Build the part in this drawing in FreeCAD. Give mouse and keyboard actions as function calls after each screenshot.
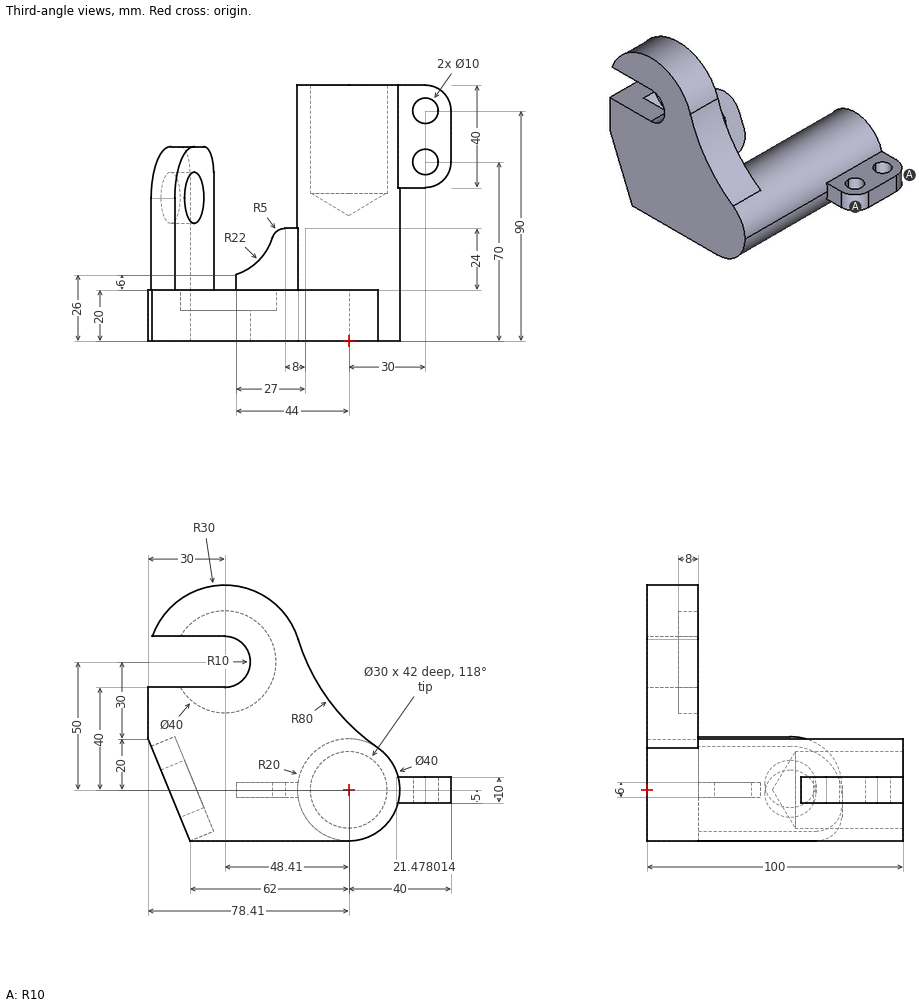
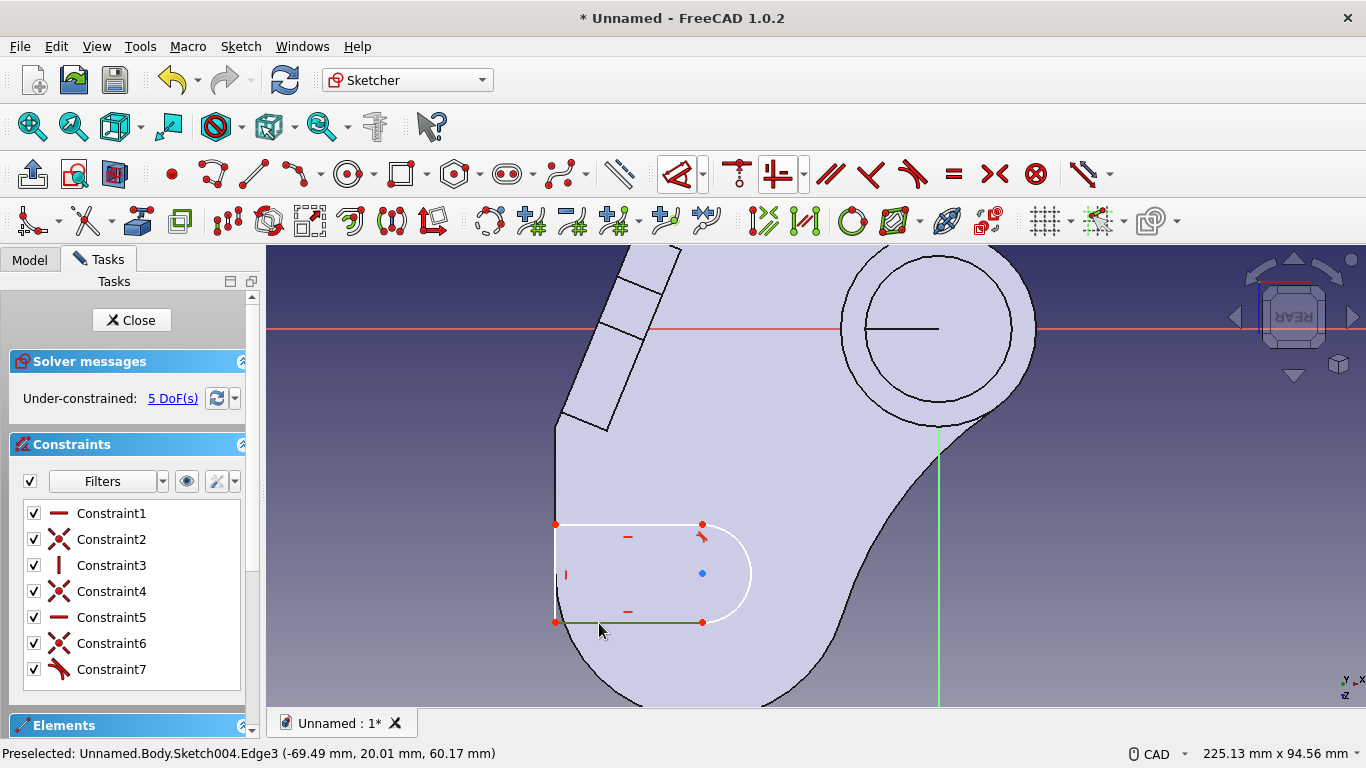
click(742, 603)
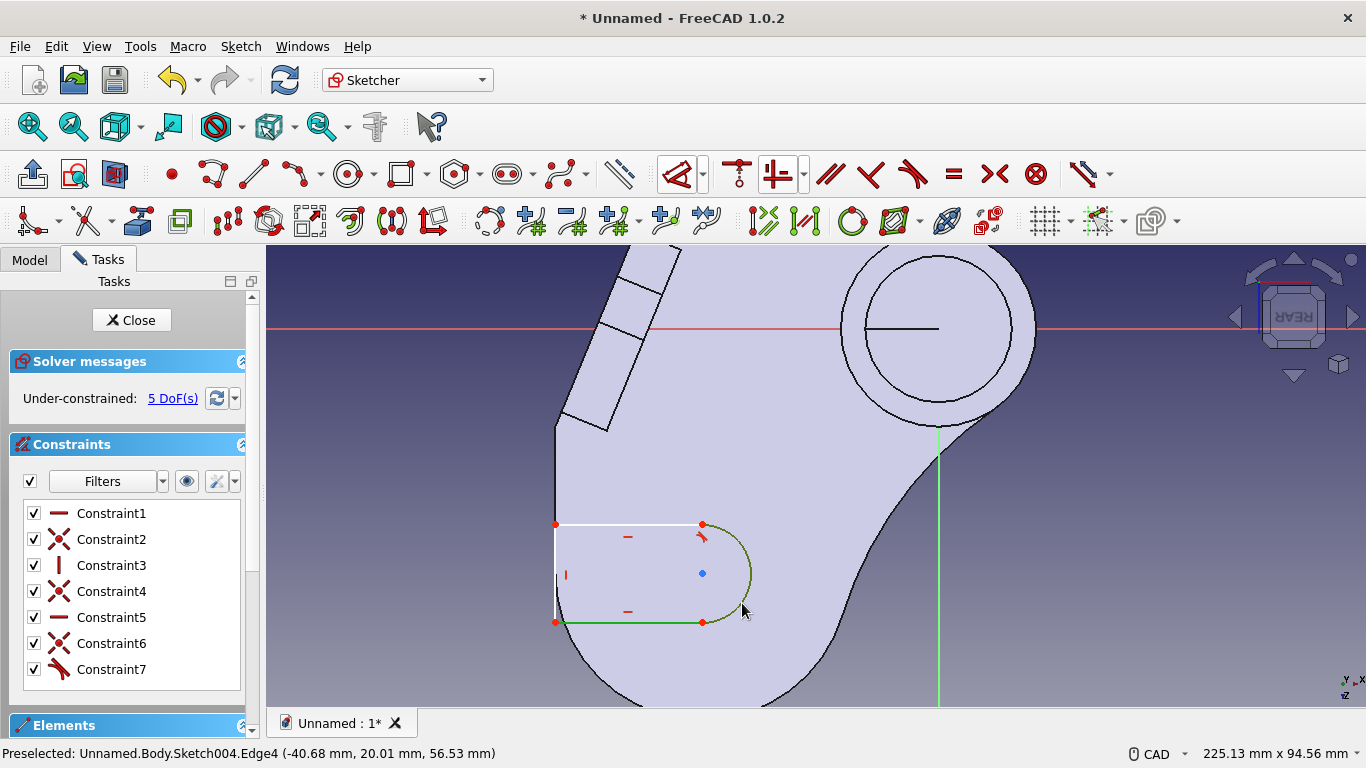
key(t)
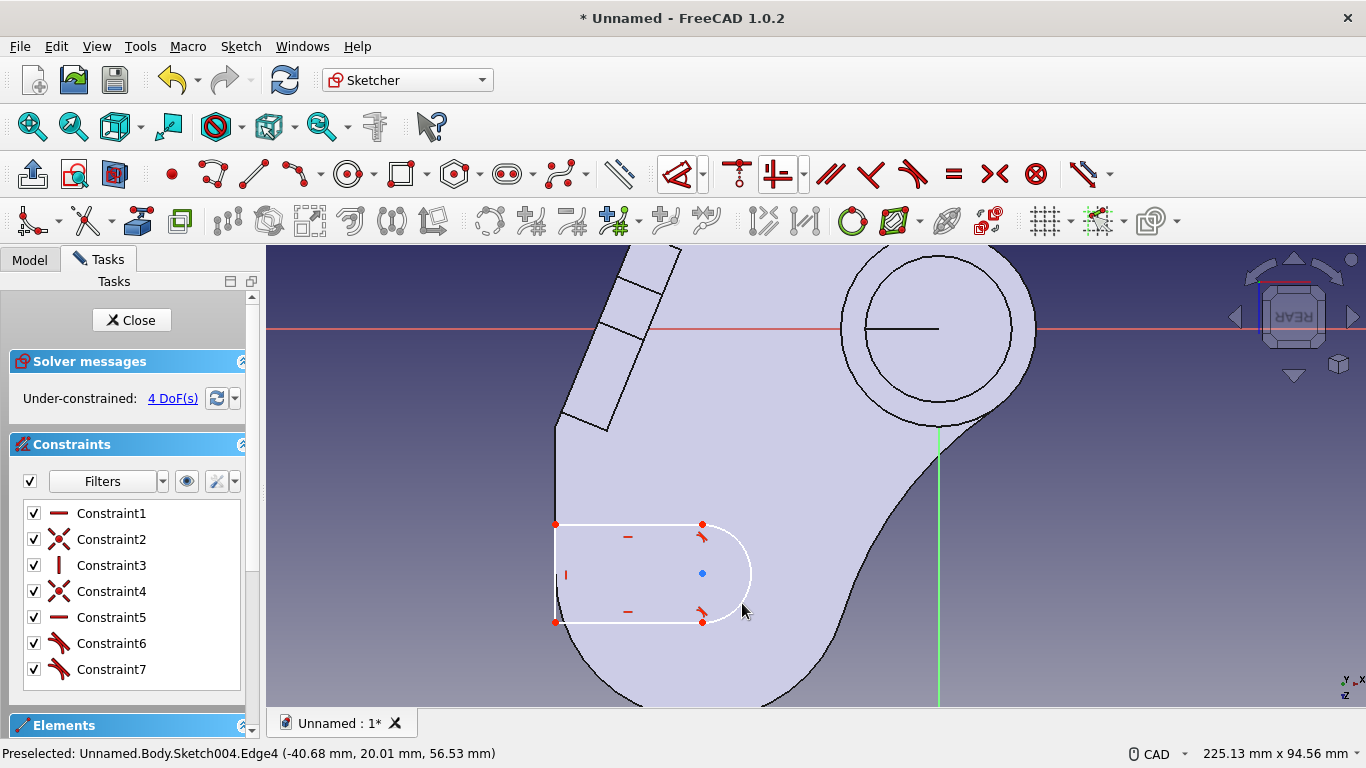
key(d)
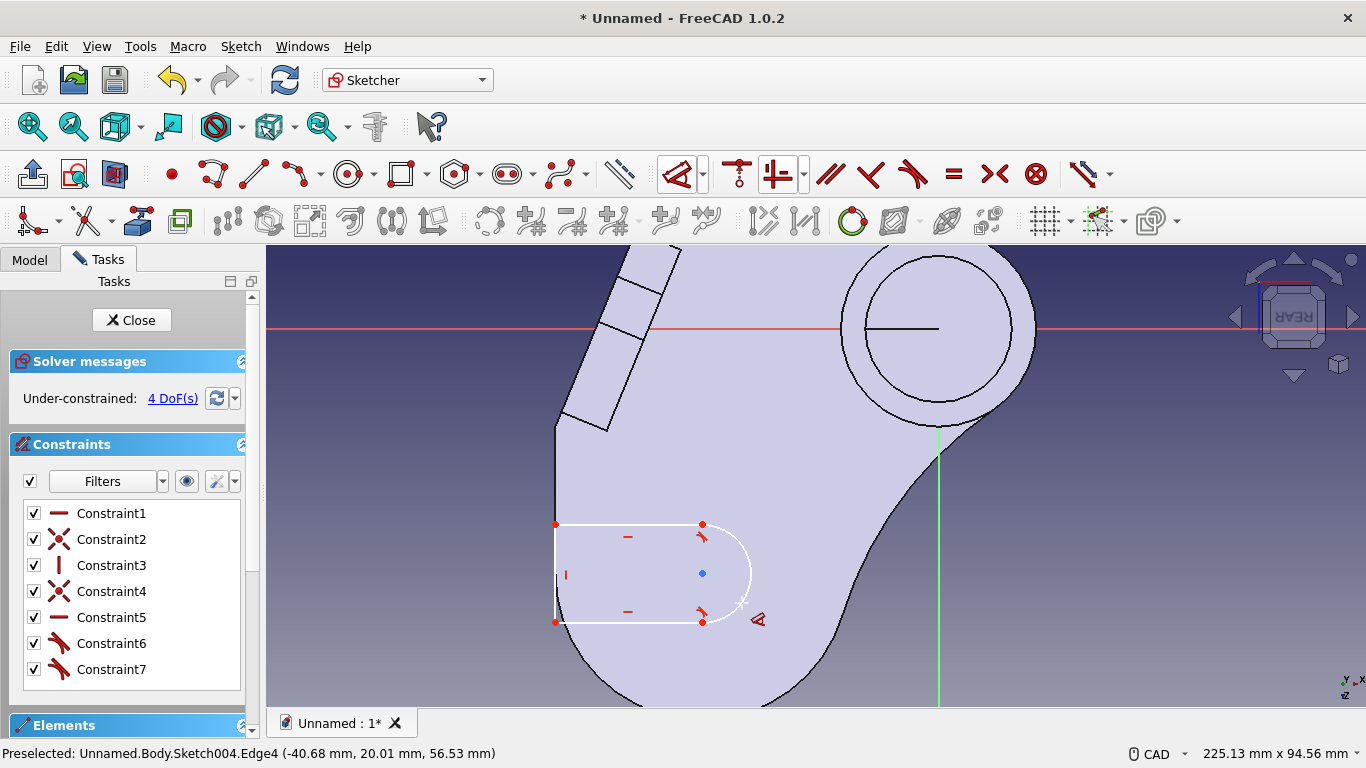
click(742, 603)
click(768, 622)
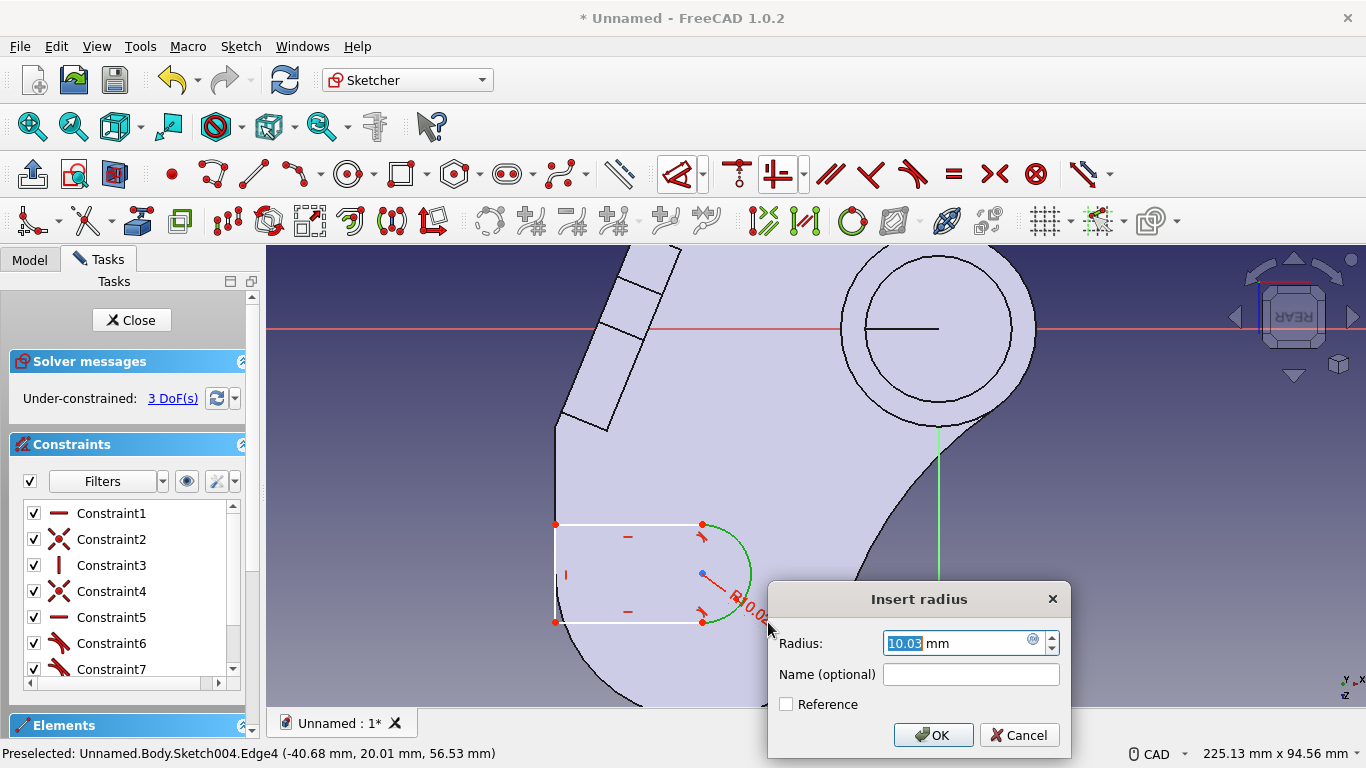
text(10)
key(Return)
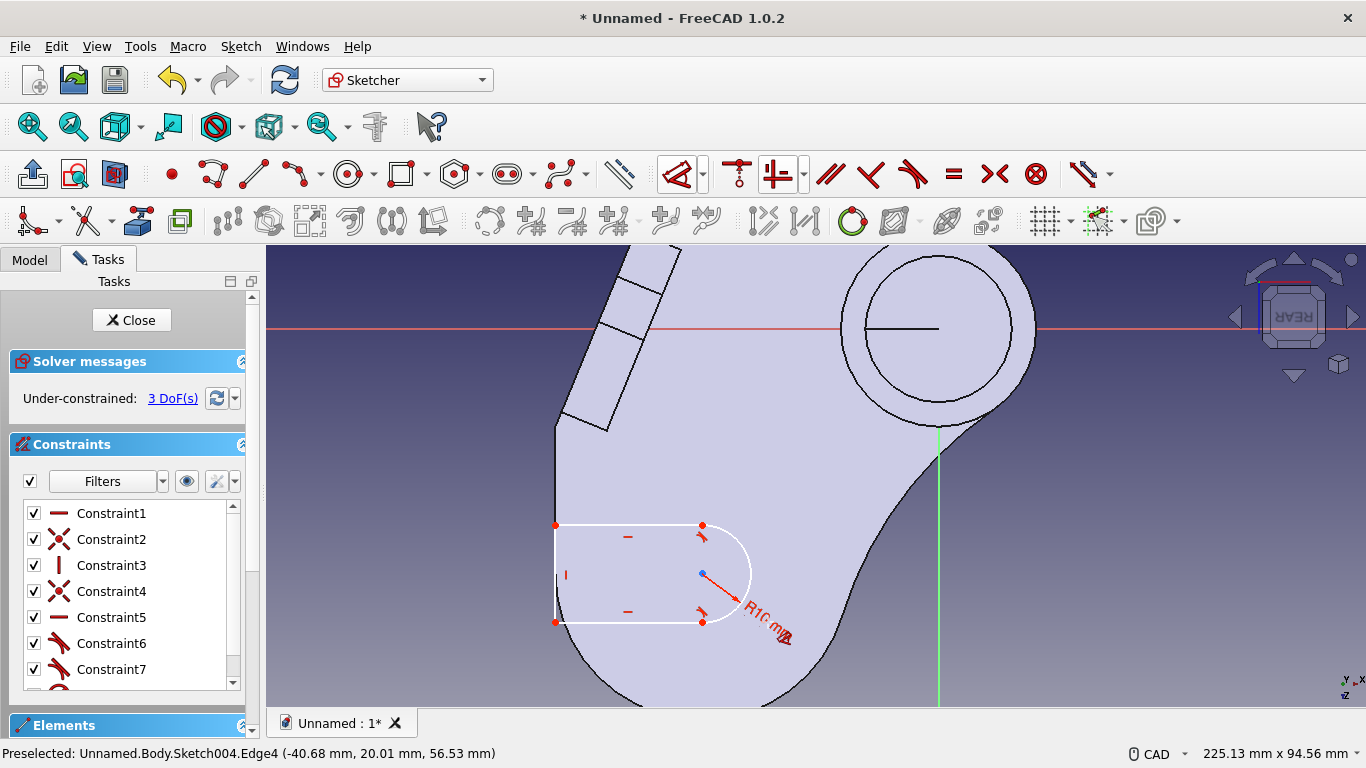
click(658, 525)
click(628, 559)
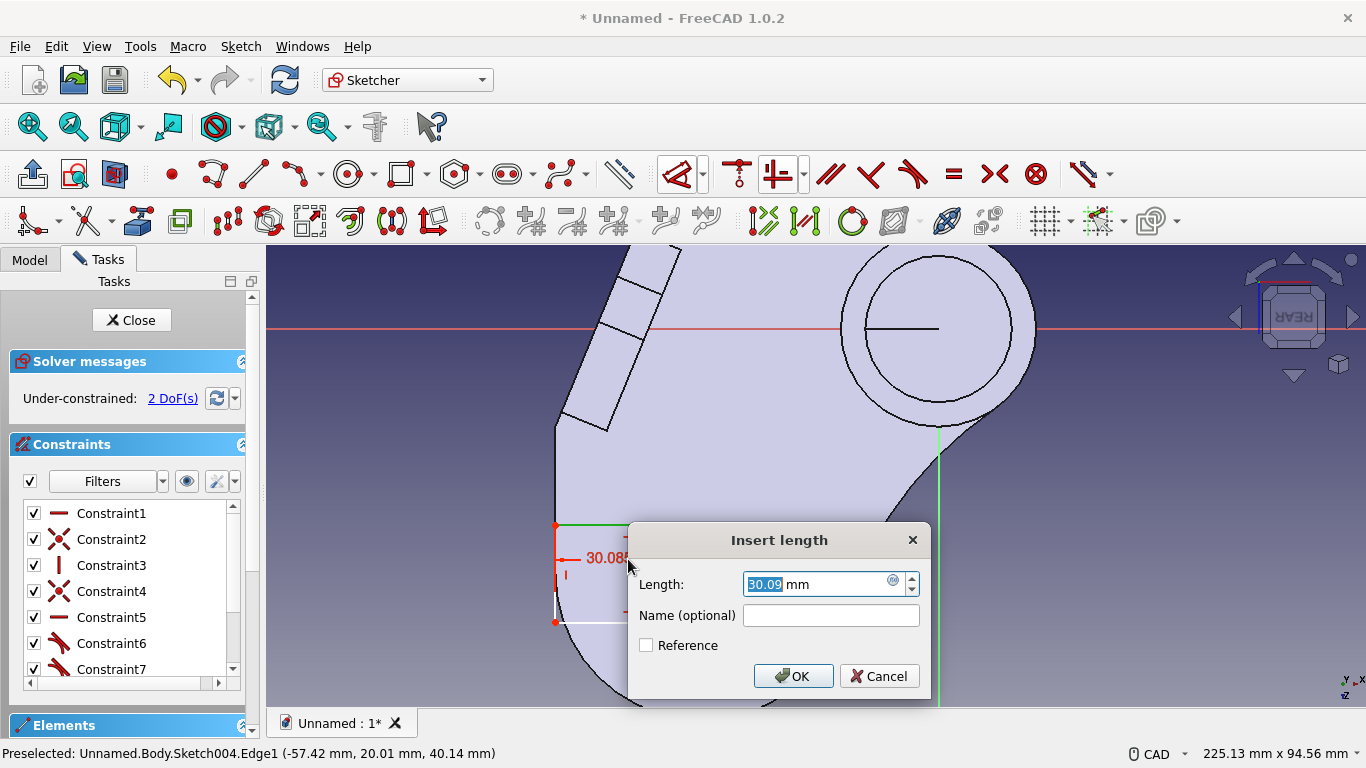
text(30)
key(Return)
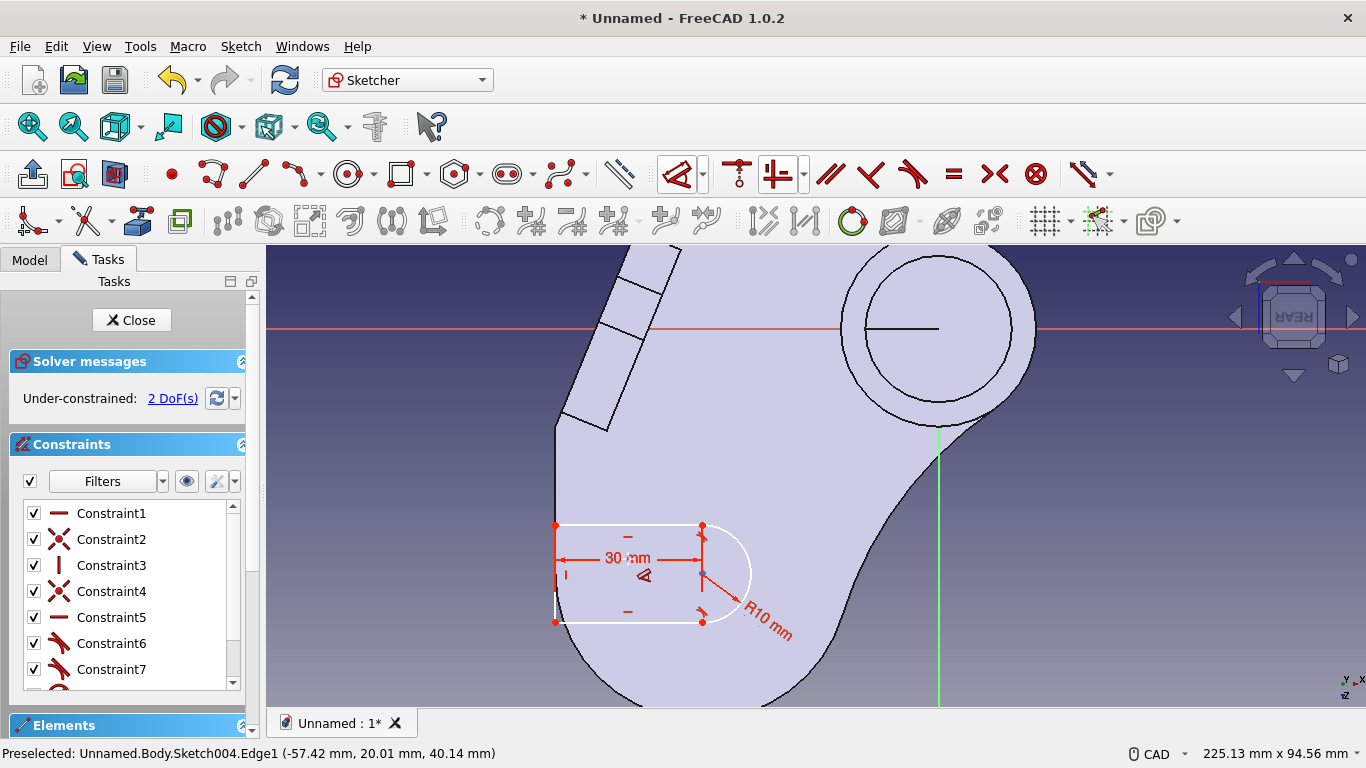
click(702, 525)
click(973, 427)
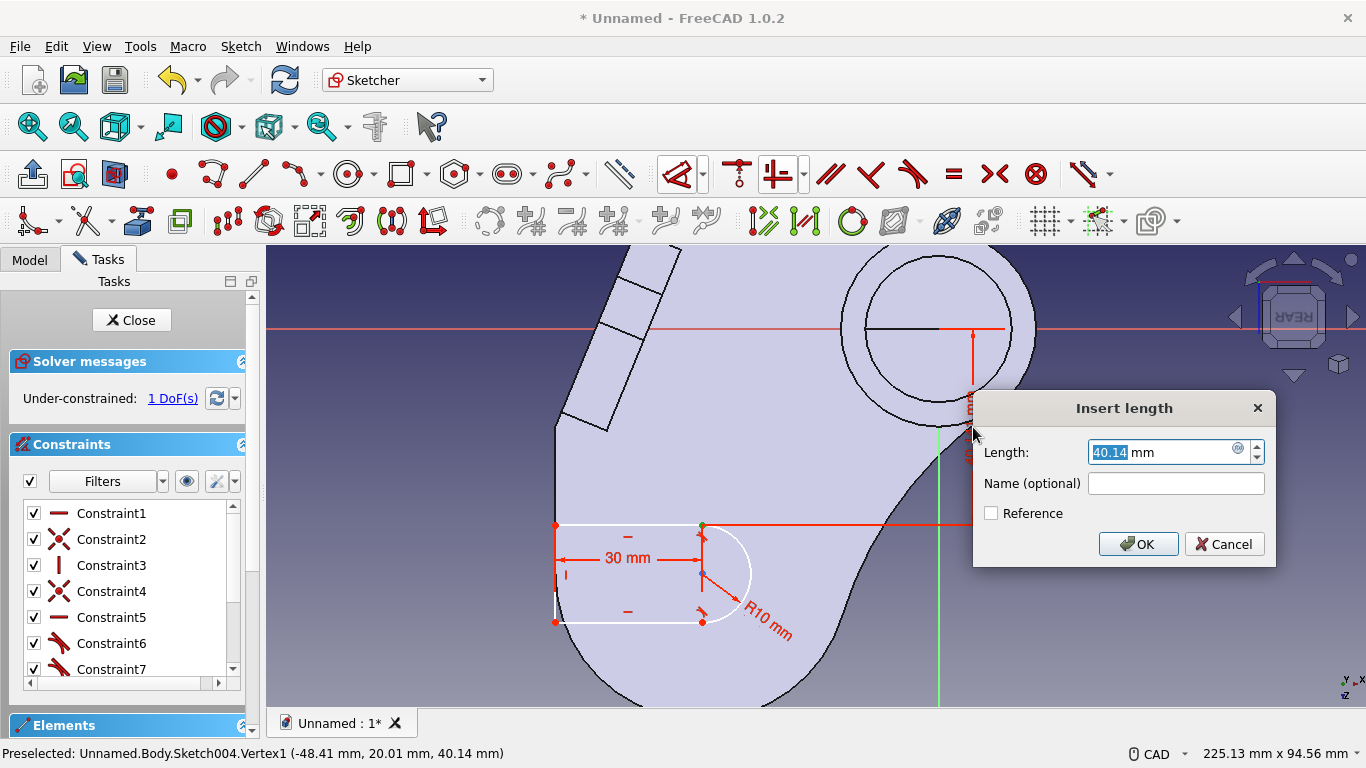
text(40)
key(Return)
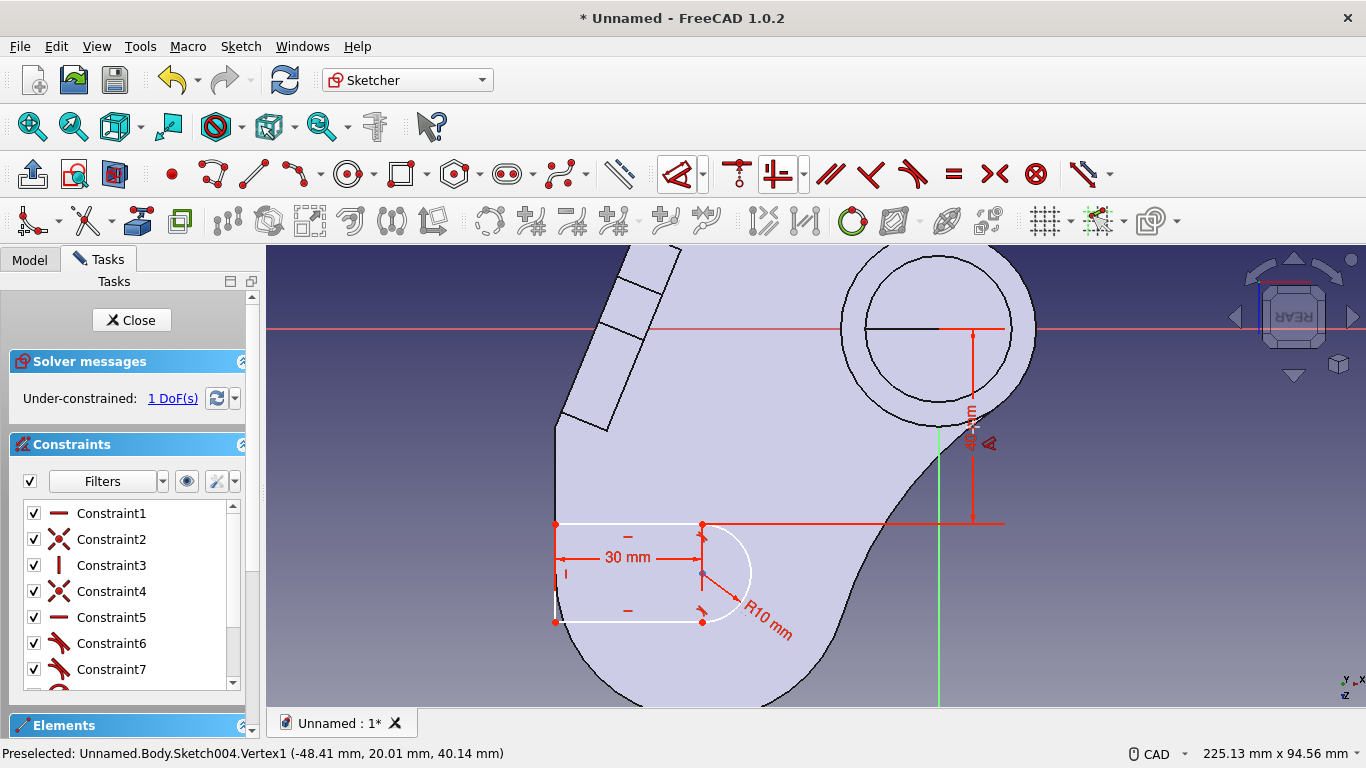
click(702, 524)
click(820, 295)